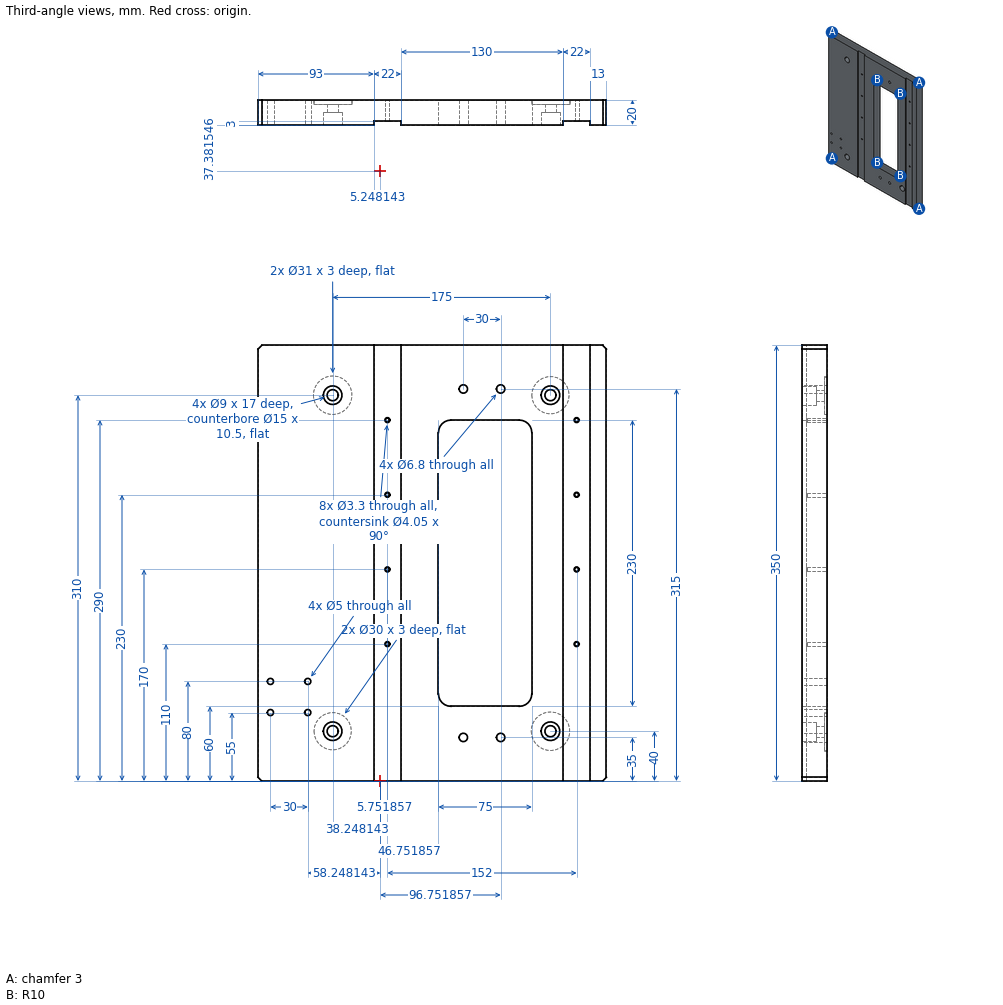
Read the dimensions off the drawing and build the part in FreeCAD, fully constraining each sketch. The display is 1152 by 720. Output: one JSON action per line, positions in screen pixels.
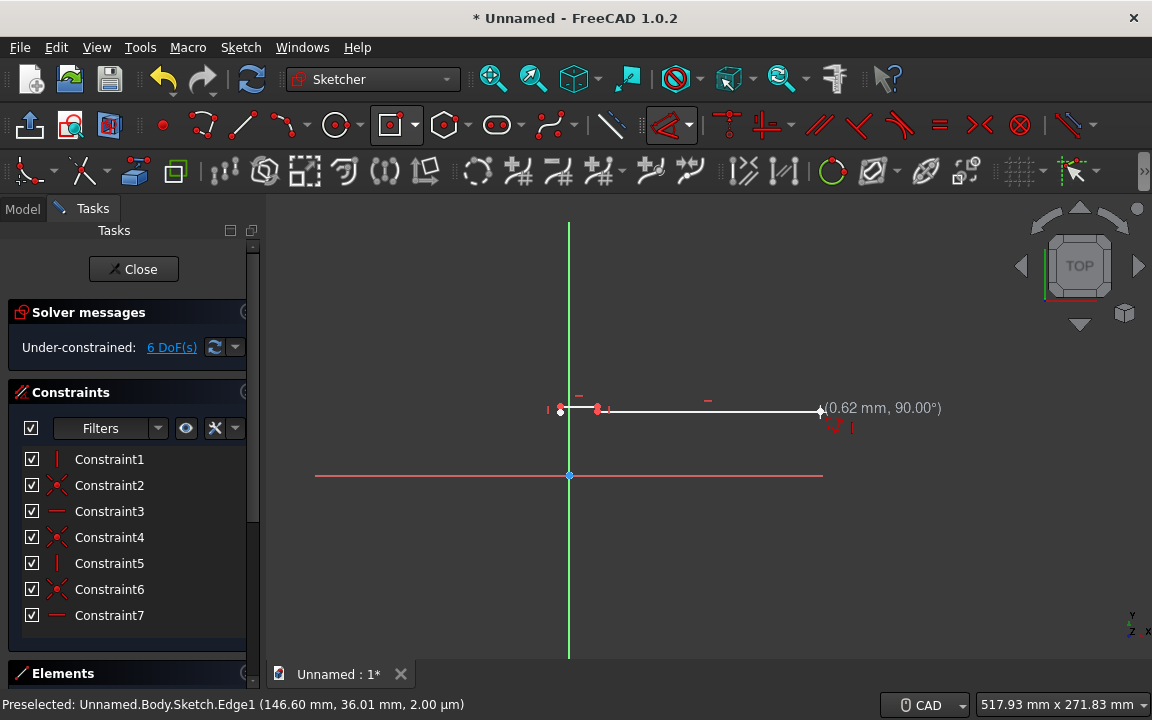
{"action": "scroll", "coordinate": [820, 407], "scroll_direction": "up", "scroll_amount": 6}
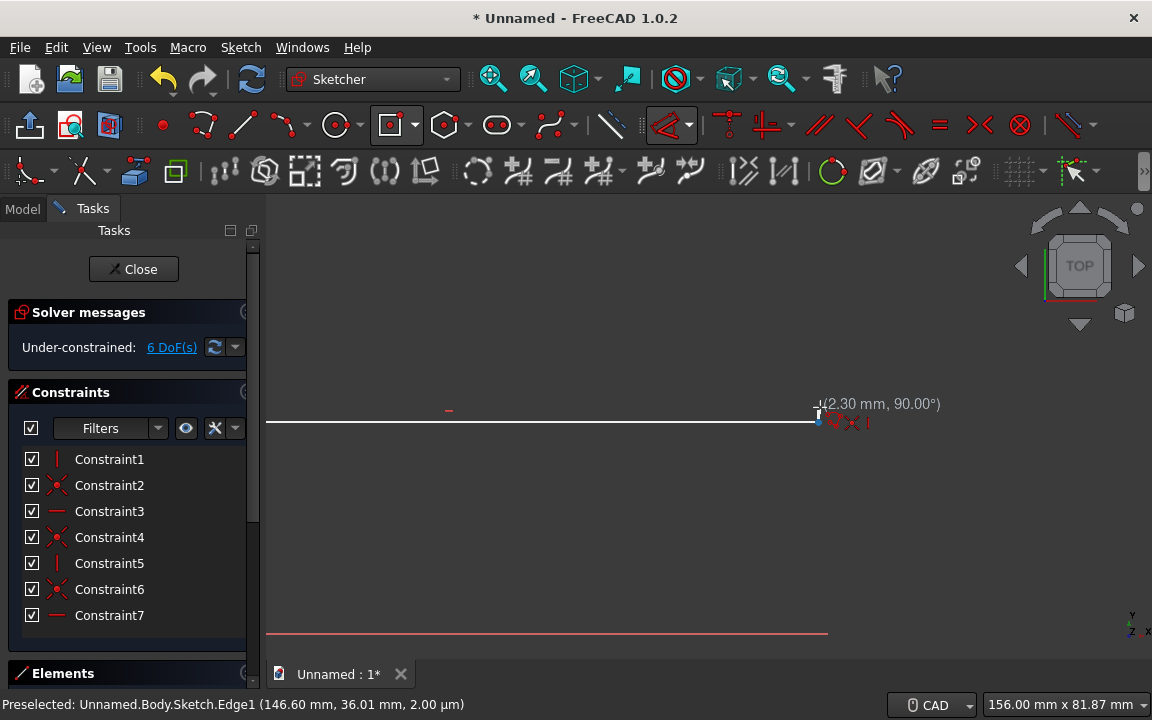
{"action": "left_click", "coordinate": [819, 404]}
{"action": "left_click", "coordinate": [944, 404]}
{"action": "left_click", "coordinate": [944, 421]}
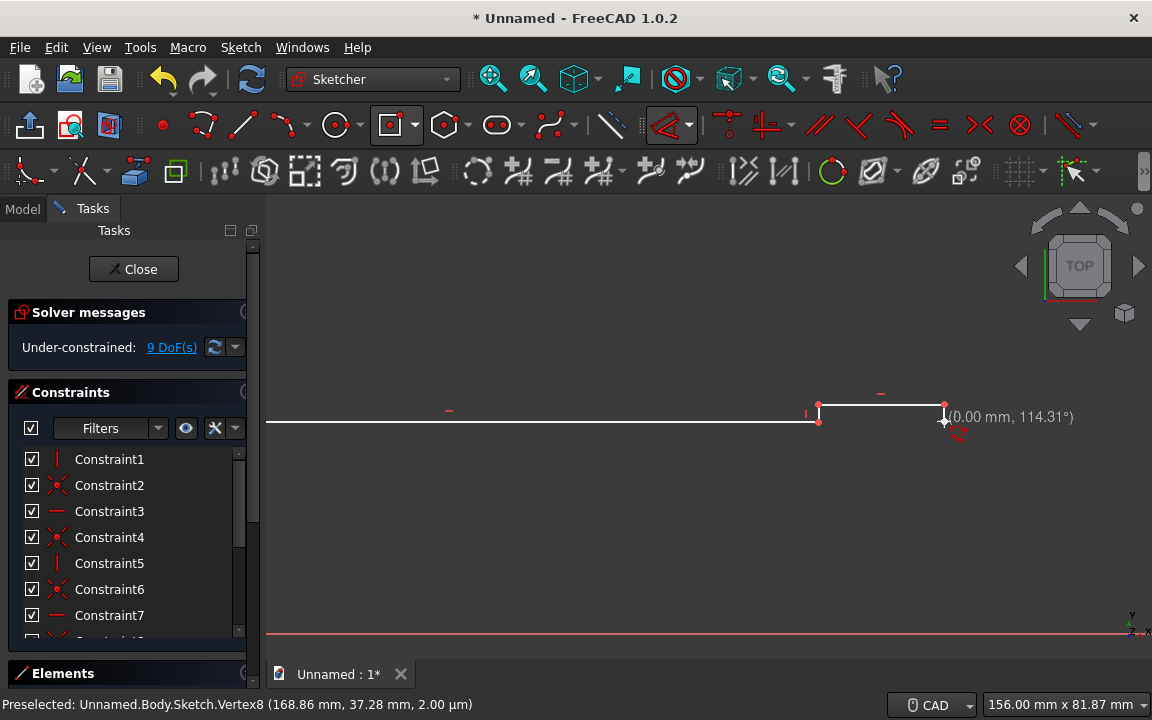
{"action": "scroll", "coordinate": [820, 407], "scroll_direction": "down", "scroll_amount": 6}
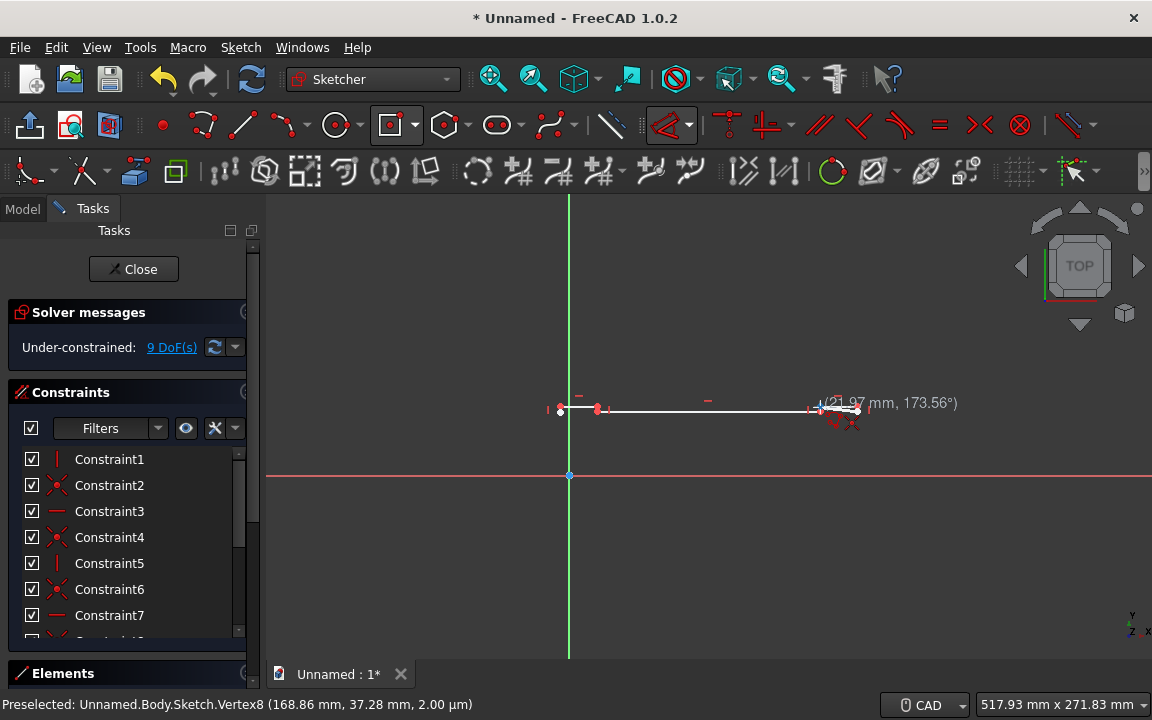
{"action": "left_click", "coordinate": [880, 412]}
{"action": "left_click", "coordinate": [880, 377]}
{"action": "left_click", "coordinate": [401, 377]}
{"action": "left_click", "coordinate": [401, 412]}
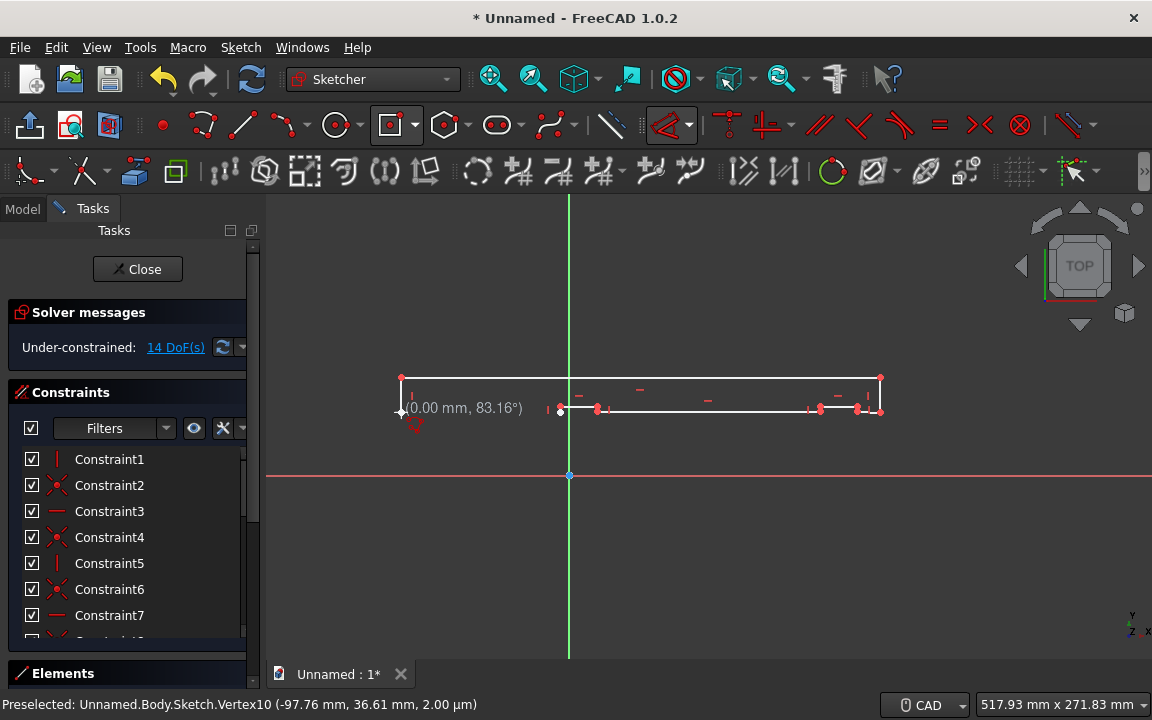
{"action": "scroll", "coordinate": [560, 412], "scroll_direction": "up", "scroll_amount": 10}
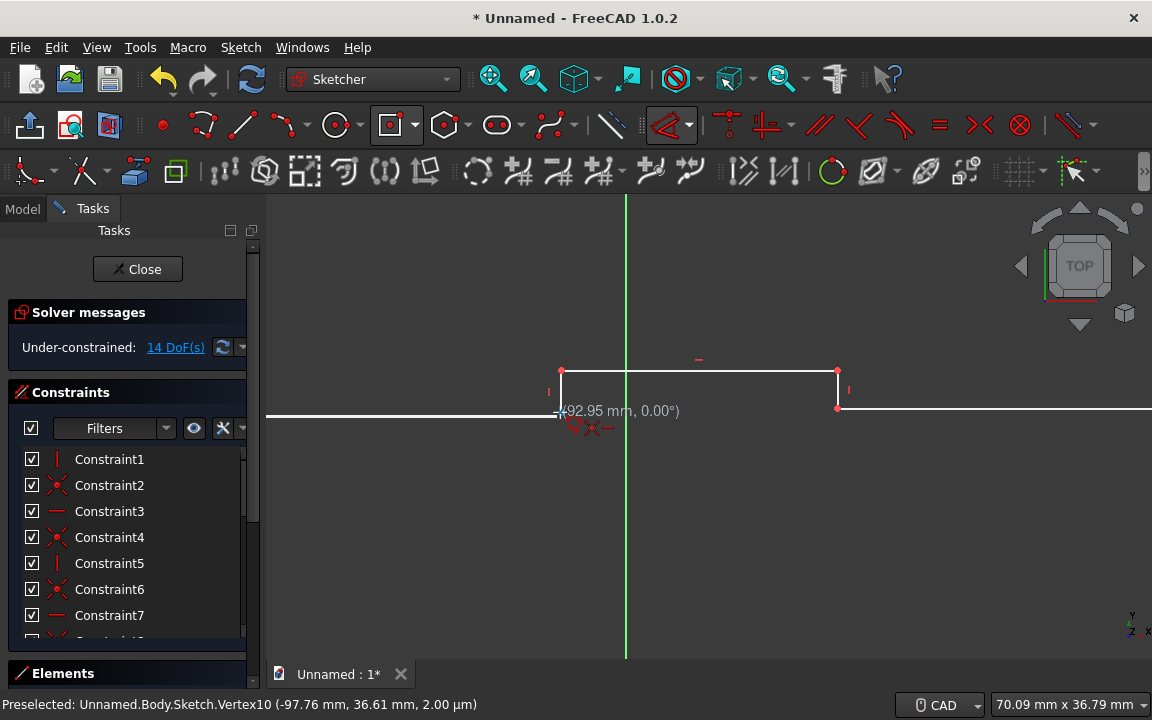
{"action": "left_click", "coordinate": [561, 412]}
{"action": "key", "text": "Escape"}
{"action": "key", "text": "Escape"}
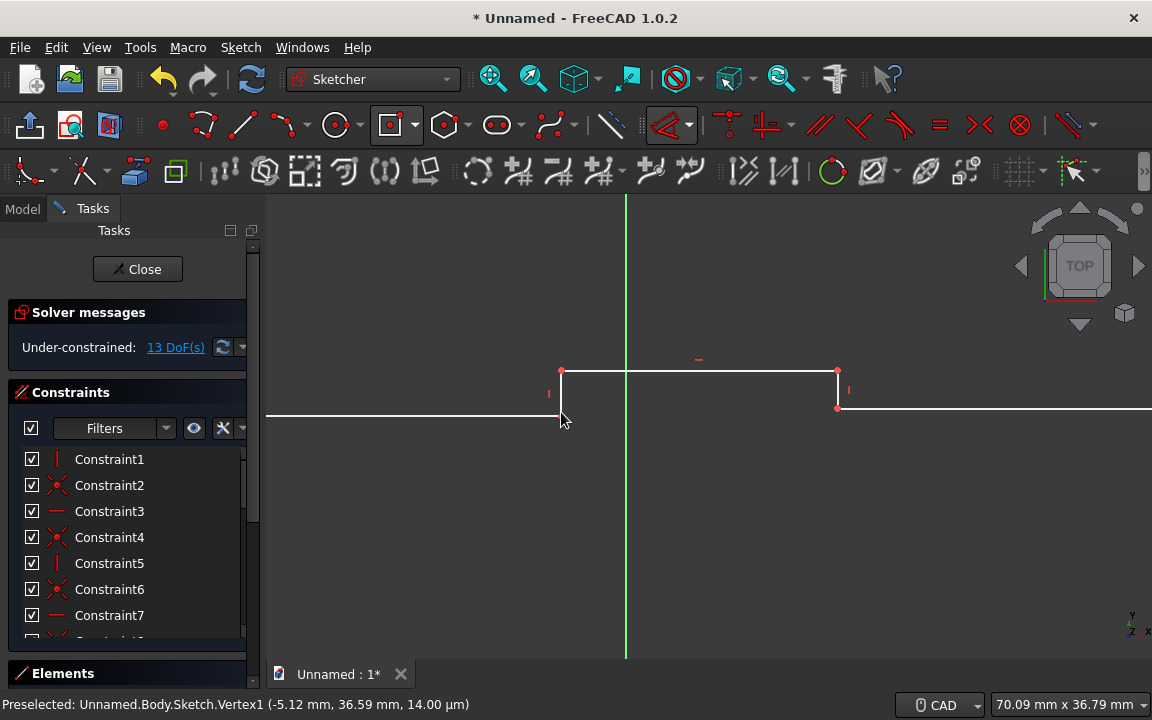
{"action": "scroll", "coordinate": [560, 412], "scroll_direction": "down", "scroll_amount": 10}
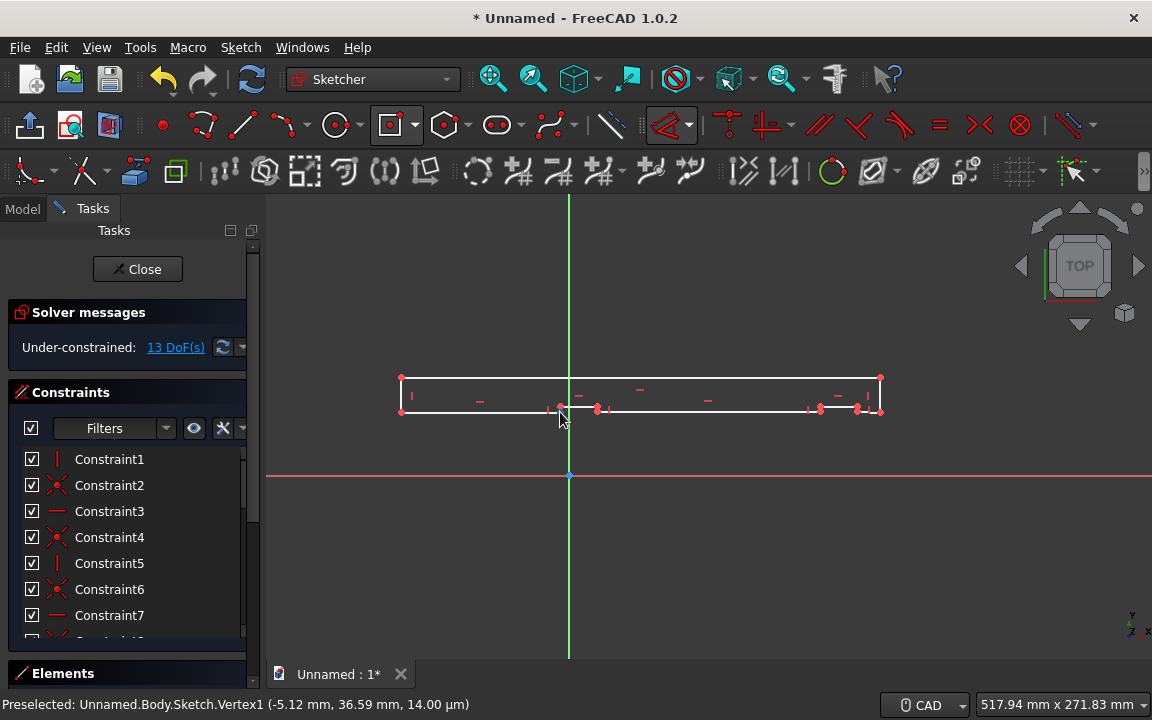
{"action": "scroll", "coordinate": [864, 412], "scroll_direction": "up", "scroll_amount": 4}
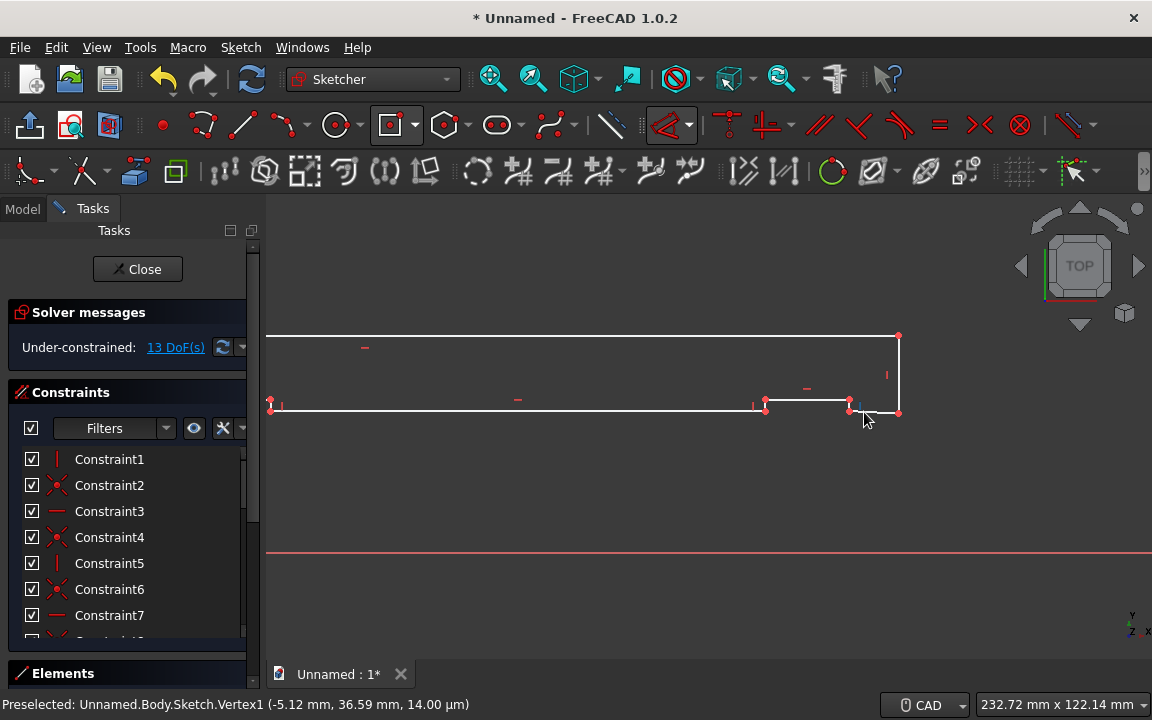
{"action": "left_click", "coordinate": [864, 412]}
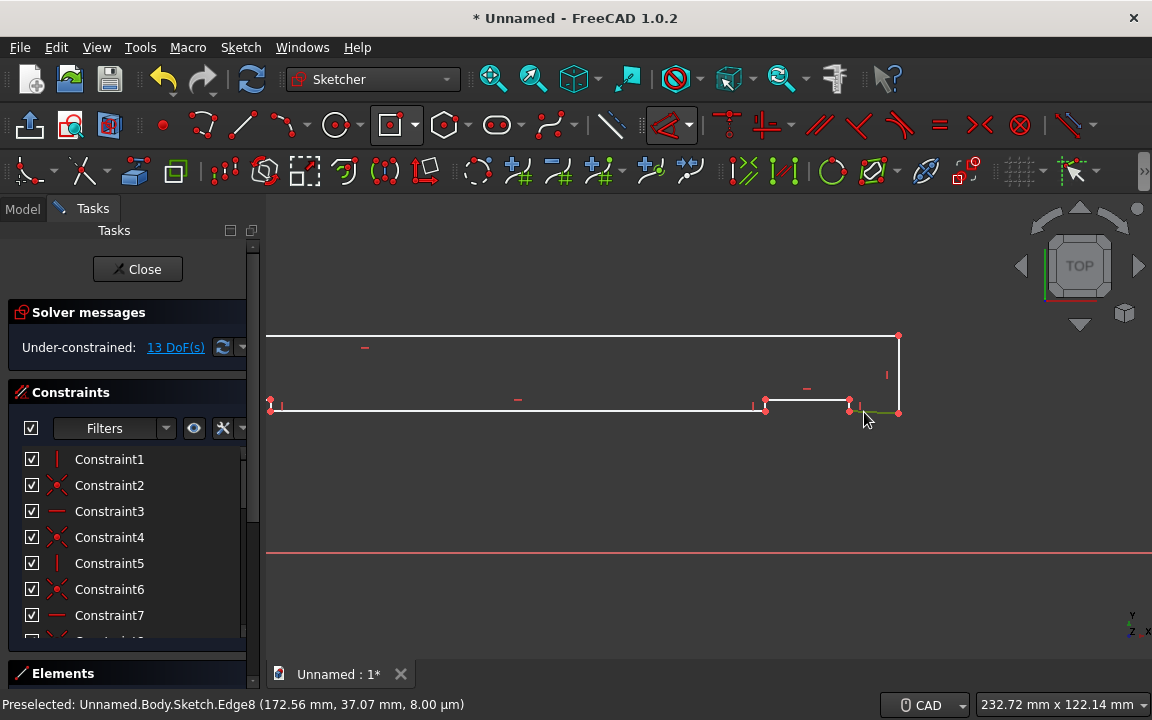
{"action": "left_click", "coordinate": [794, 126]}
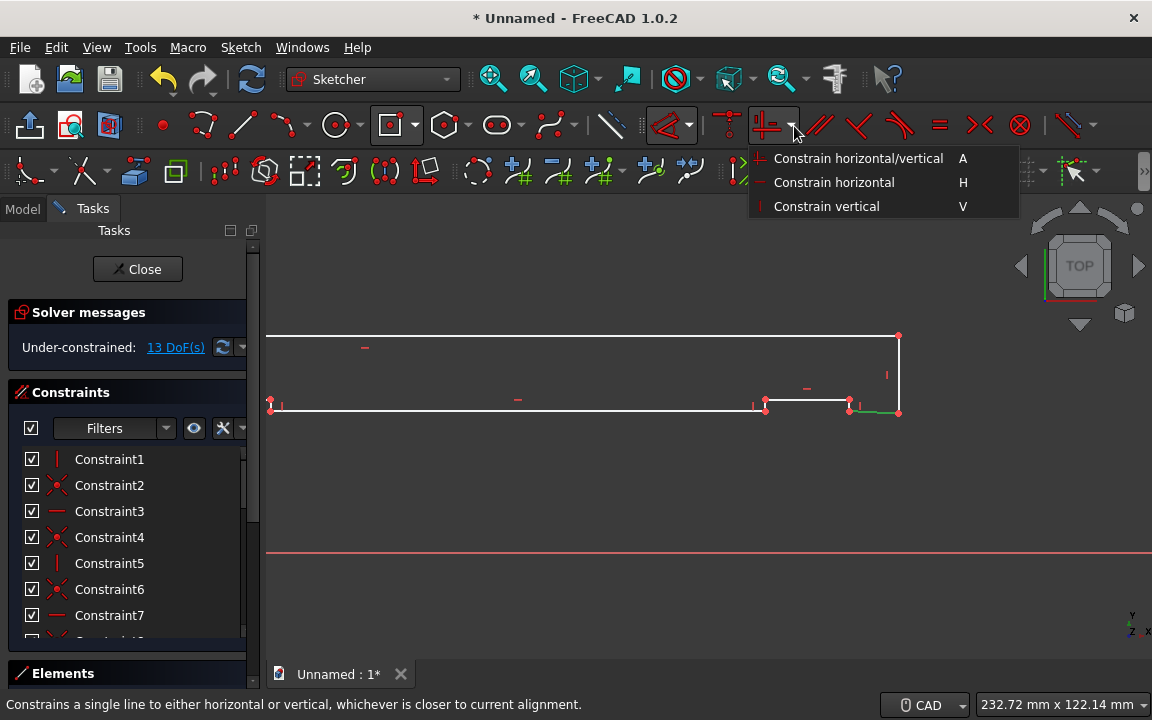
{"action": "left_click", "coordinate": [884, 182]}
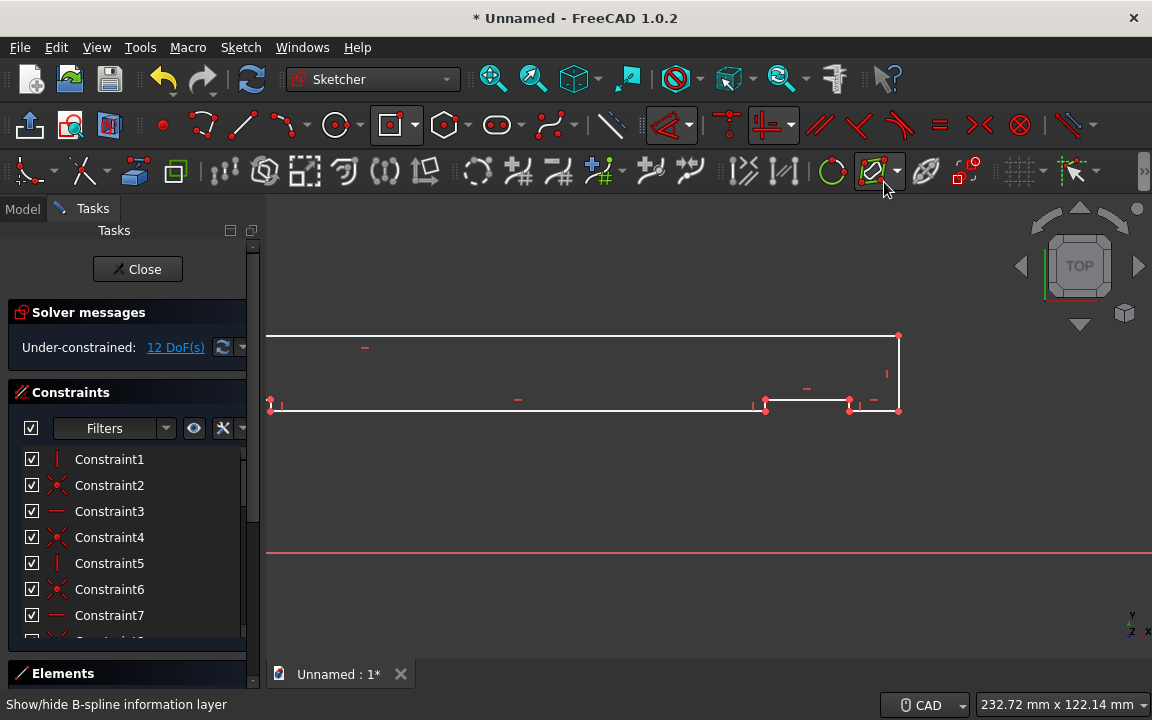
{"action": "left_click", "coordinate": [666, 126]}